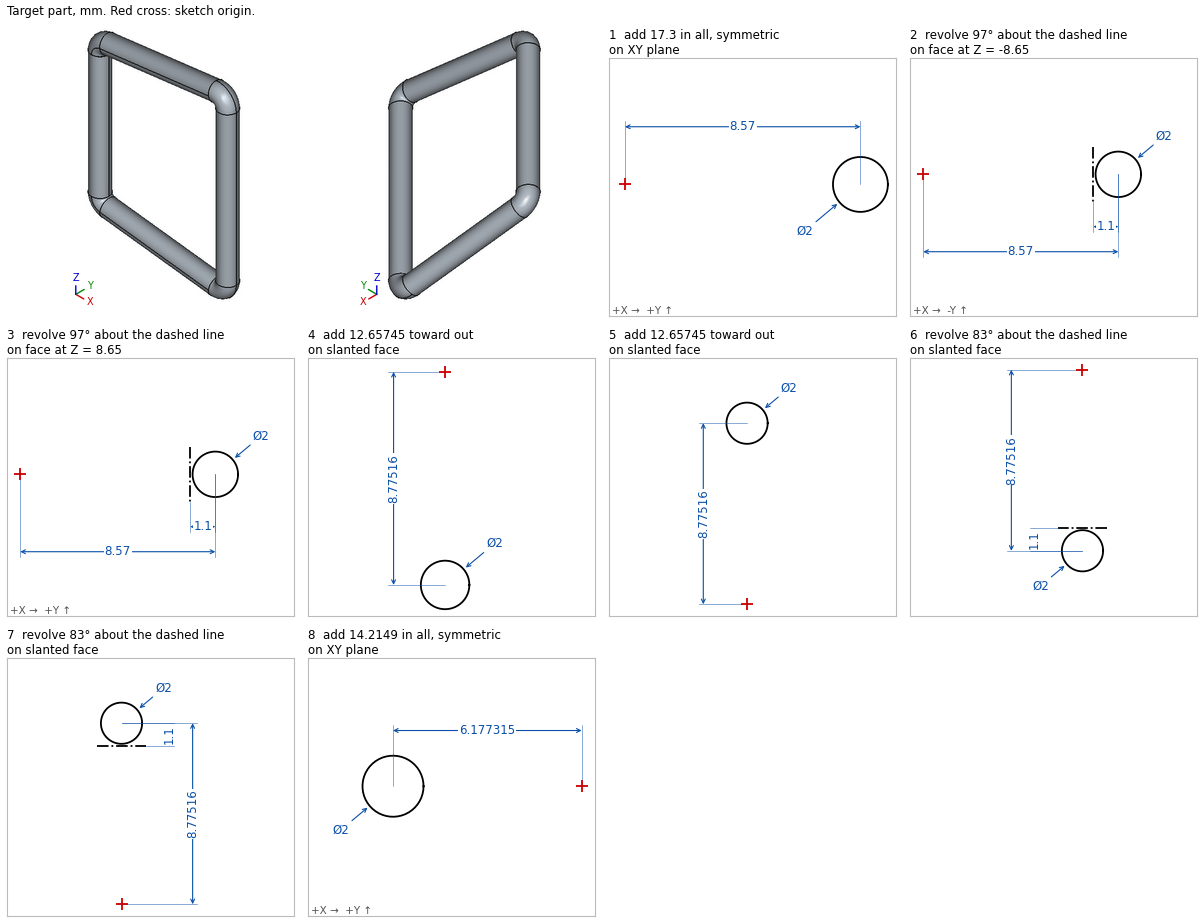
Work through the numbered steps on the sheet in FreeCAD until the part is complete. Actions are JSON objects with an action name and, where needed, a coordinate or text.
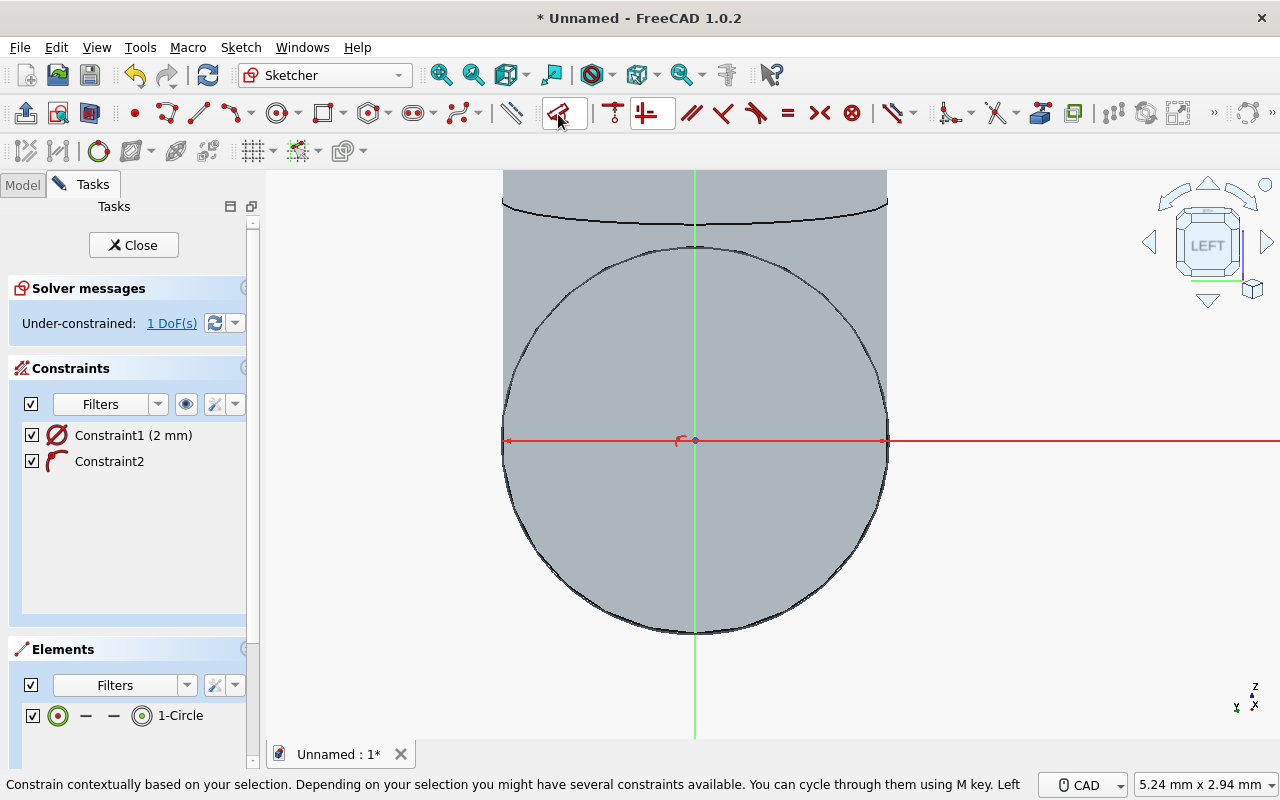
{"action": "left_click", "coordinate": [695, 441]}
{"action": "left_click", "coordinate": [661, 319]}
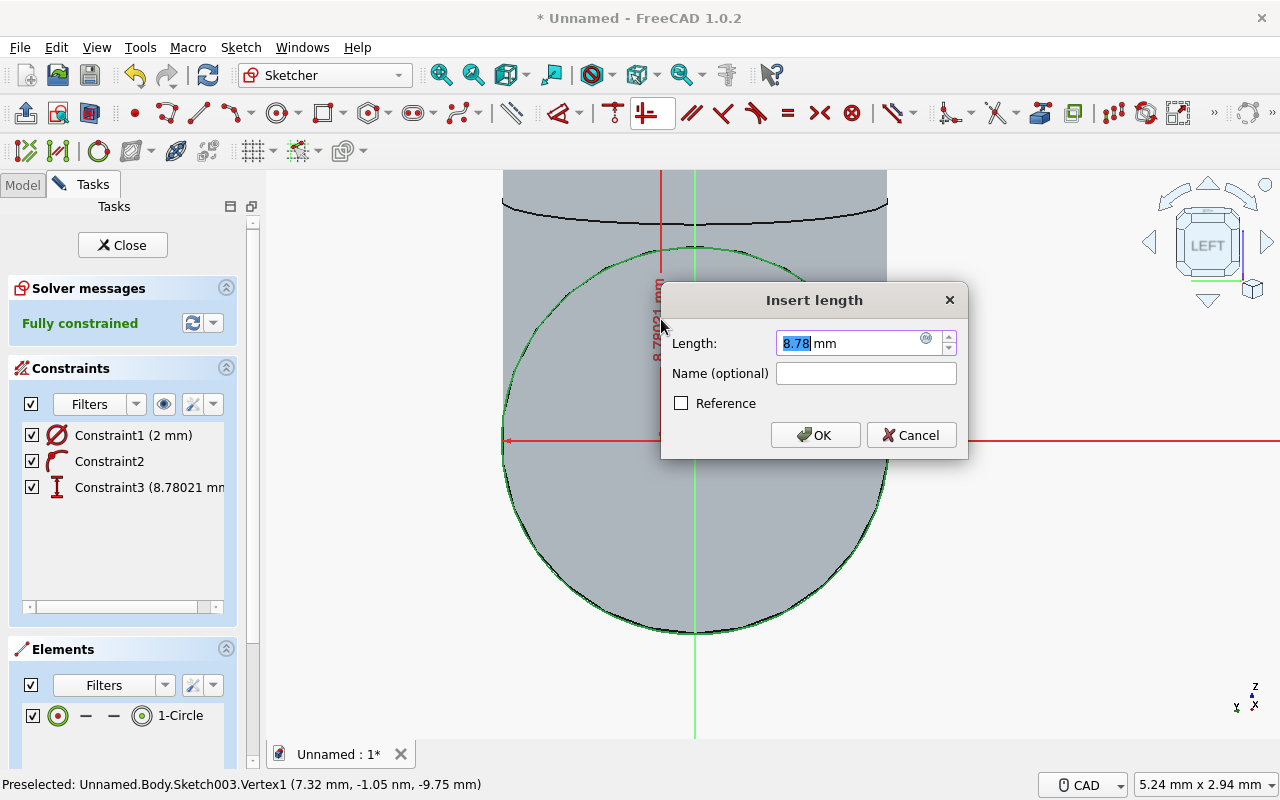
{"action": "type", "text": "8.77516"}
{"action": "key", "text": "Return"}
{"action": "key", "text": "Escape"}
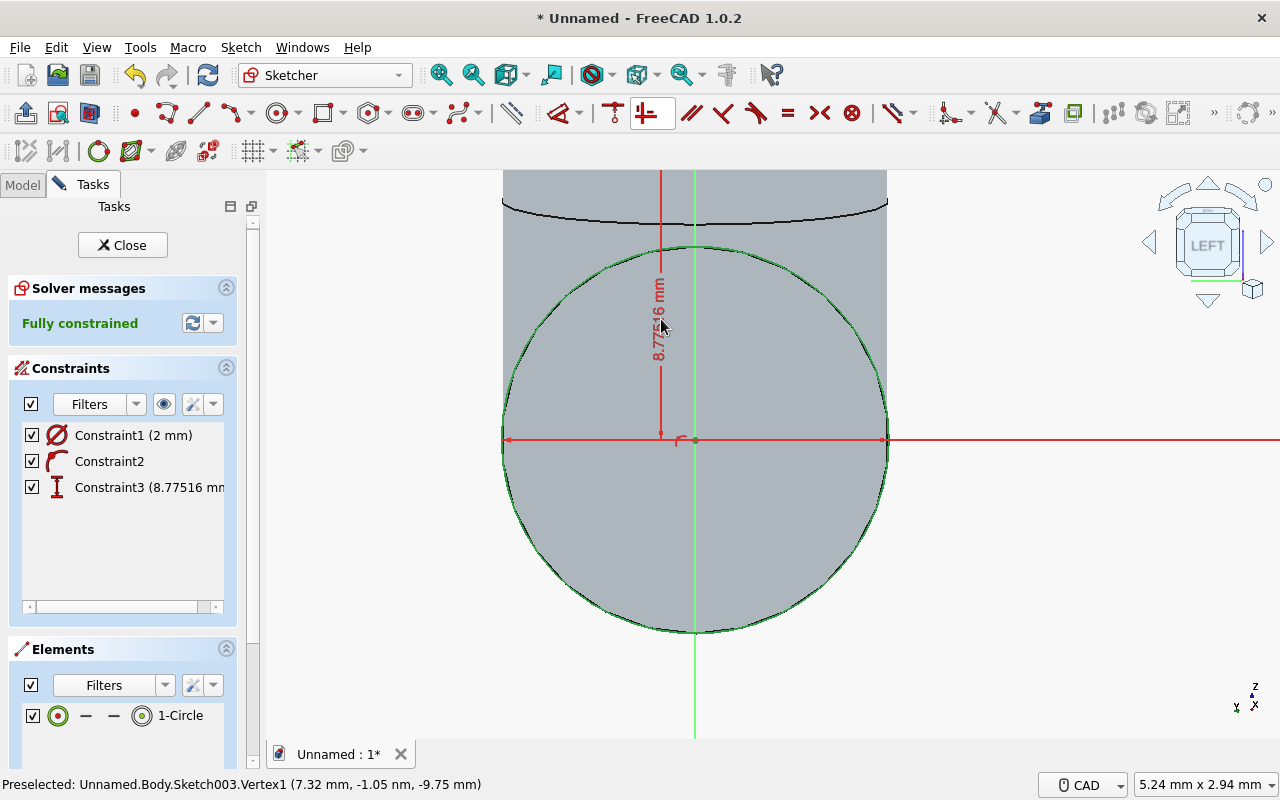
{"action": "left_click", "coordinate": [123, 245]}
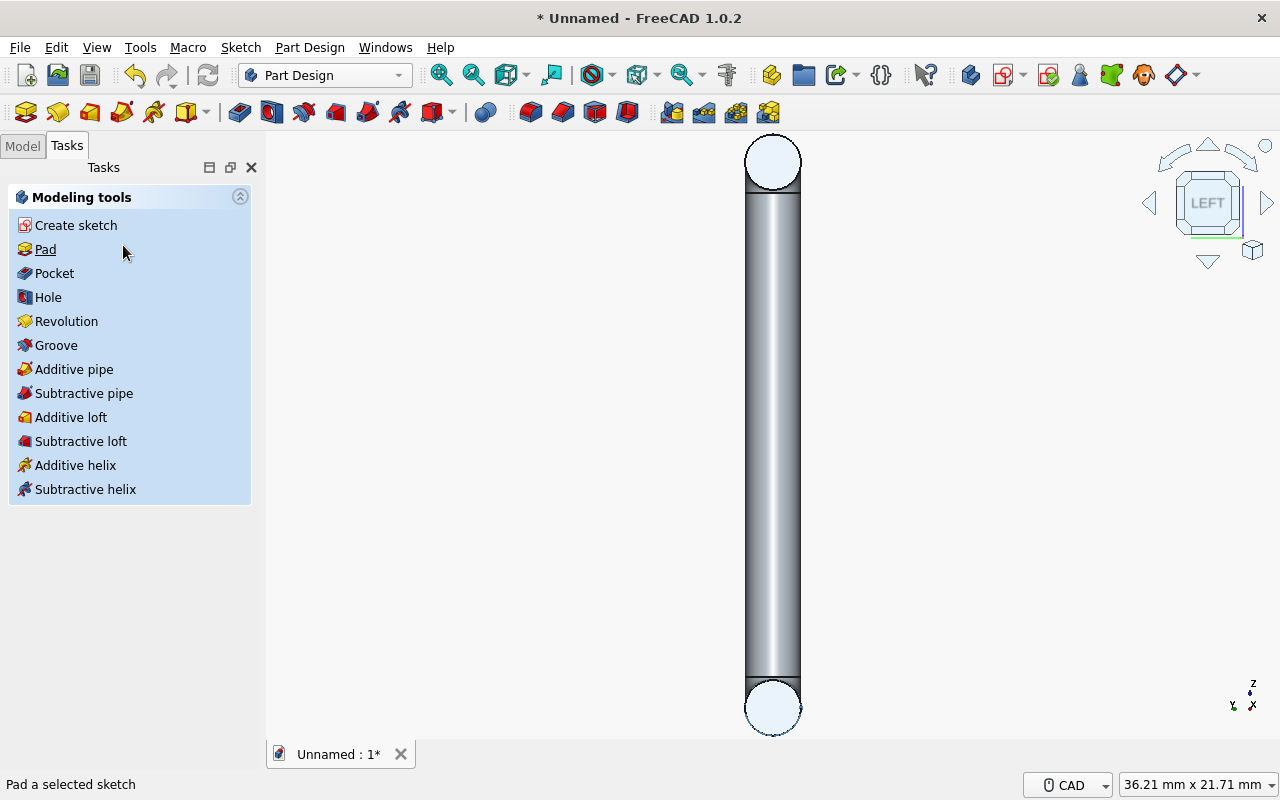
{"action": "left_click", "coordinate": [26, 112]}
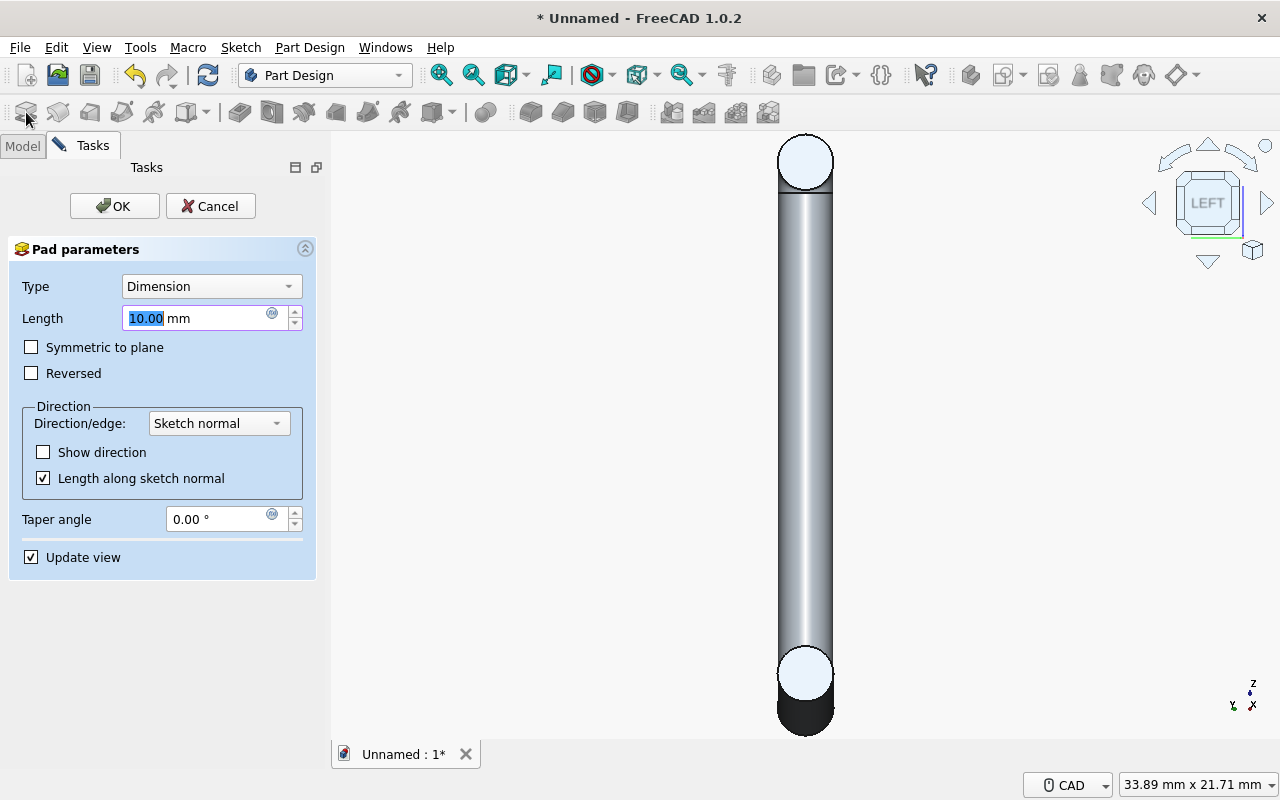
{"action": "type", "text": "12.65745"}
{"action": "key", "text": "Tab"}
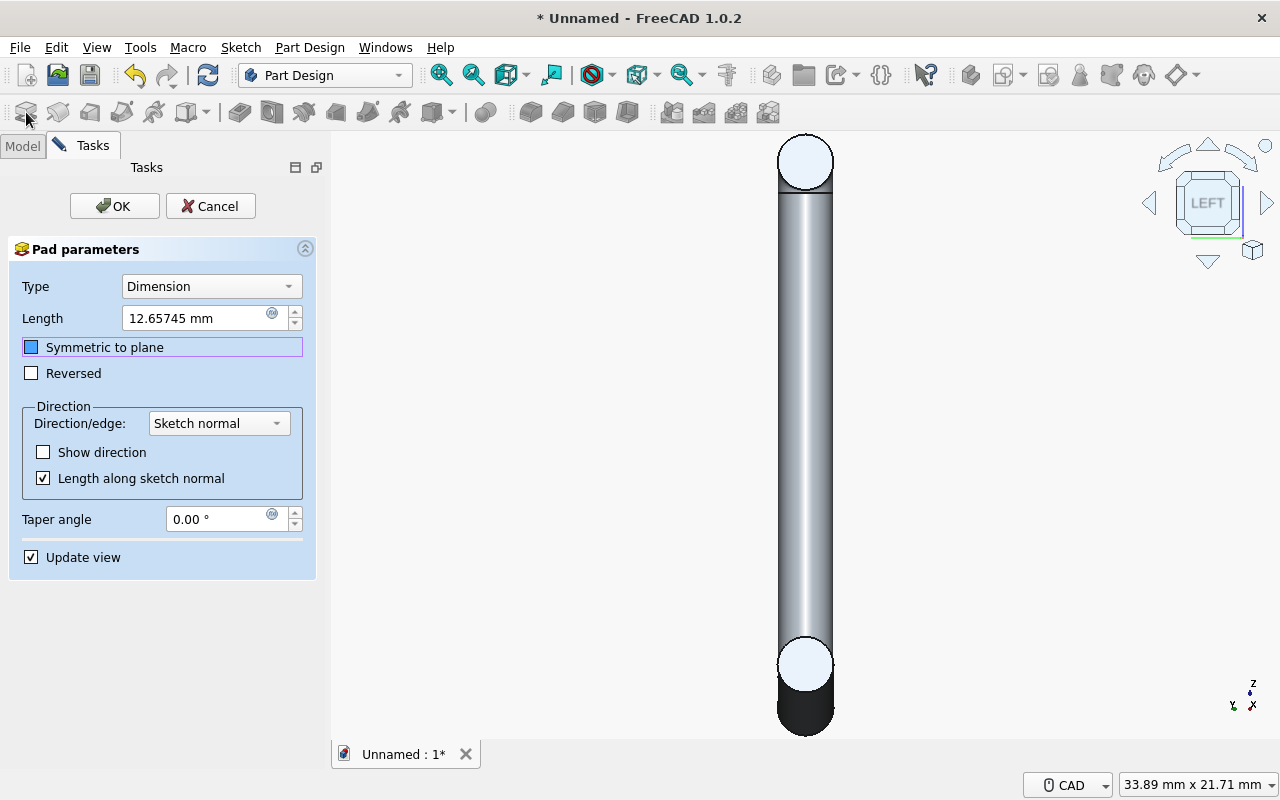
{"action": "left_click", "coordinate": [115, 206]}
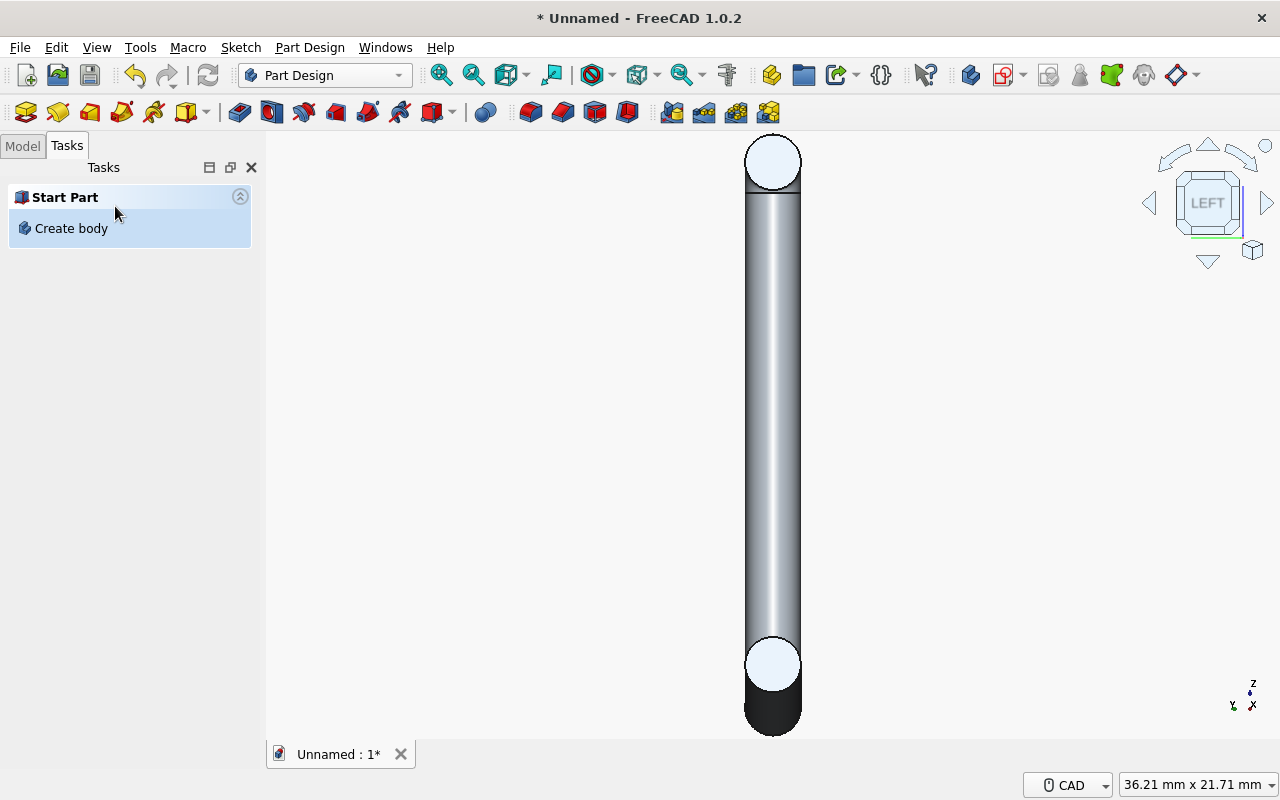
{"action": "left_click", "coordinate": [773, 161]}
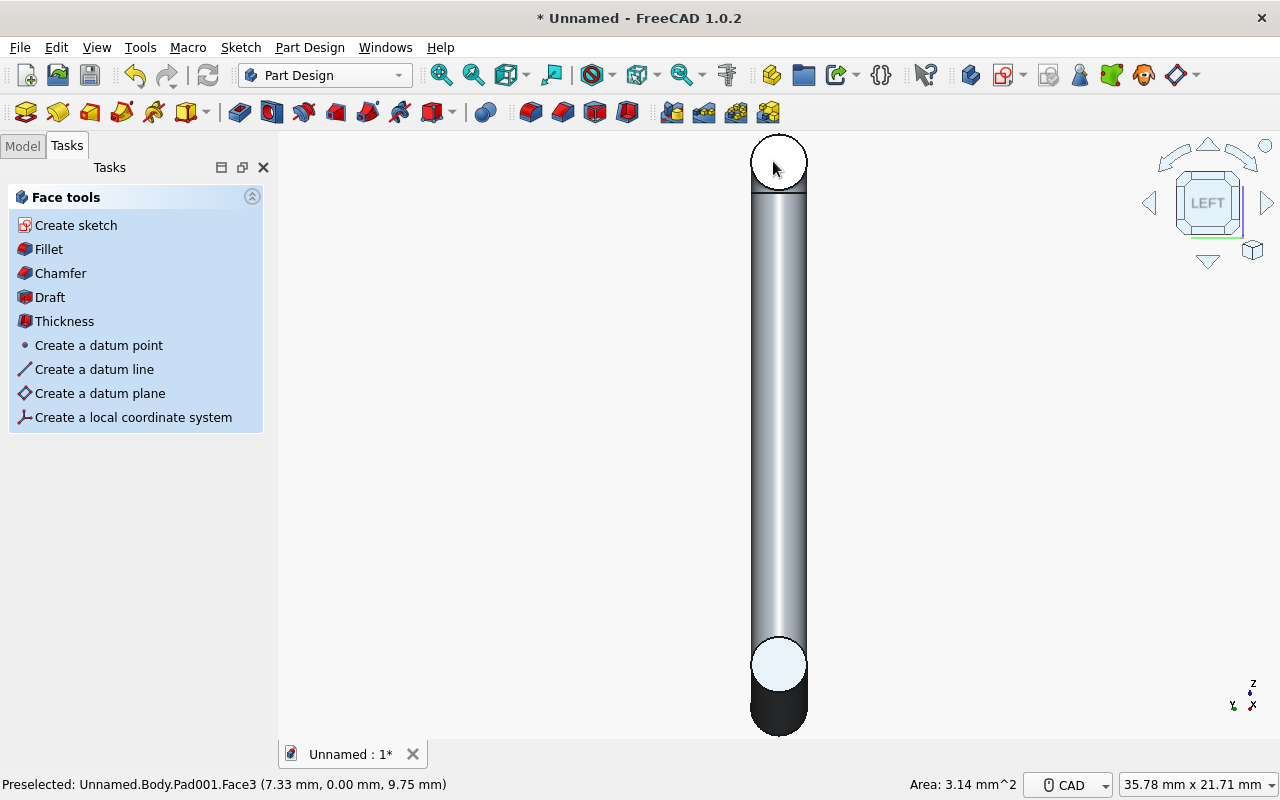
{"action": "left_click", "coordinate": [1004, 76]}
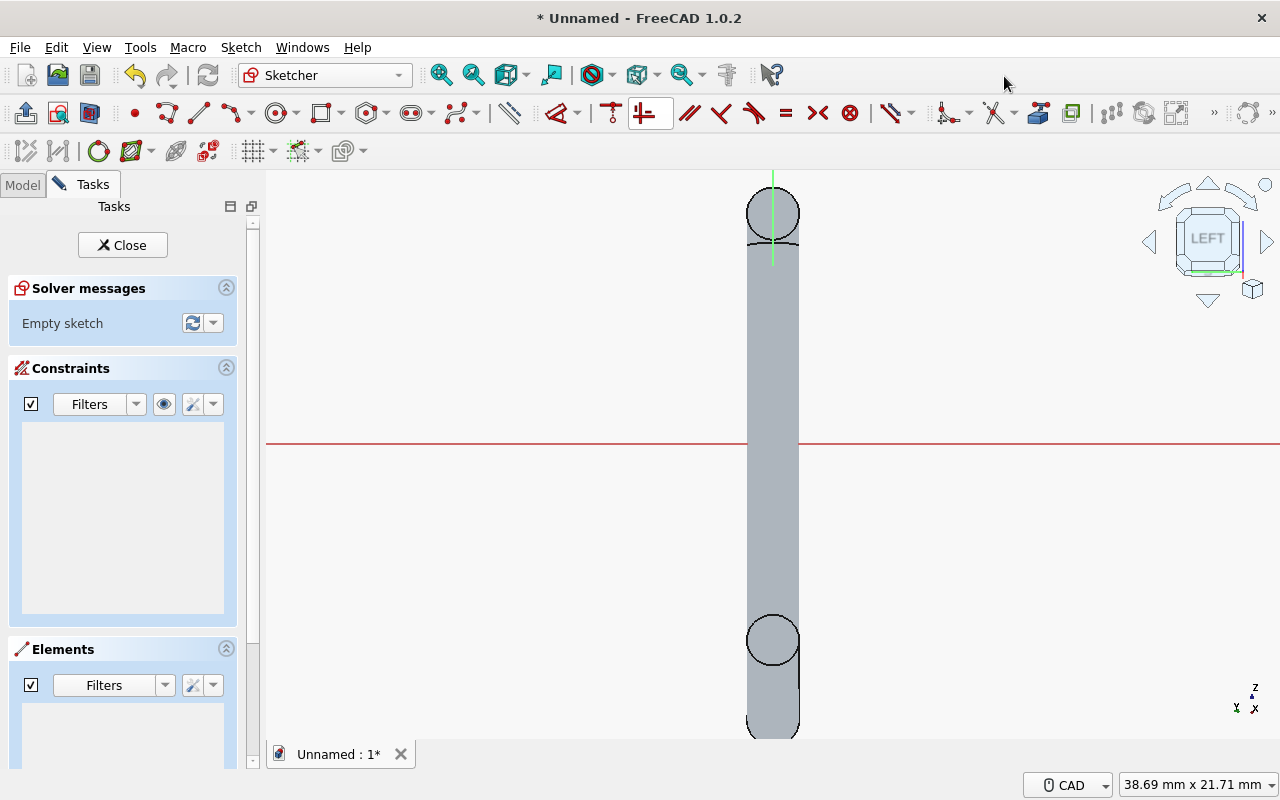
{"action": "scroll", "coordinate": [704, 454], "scroll_direction": "down", "scroll_amount": 5}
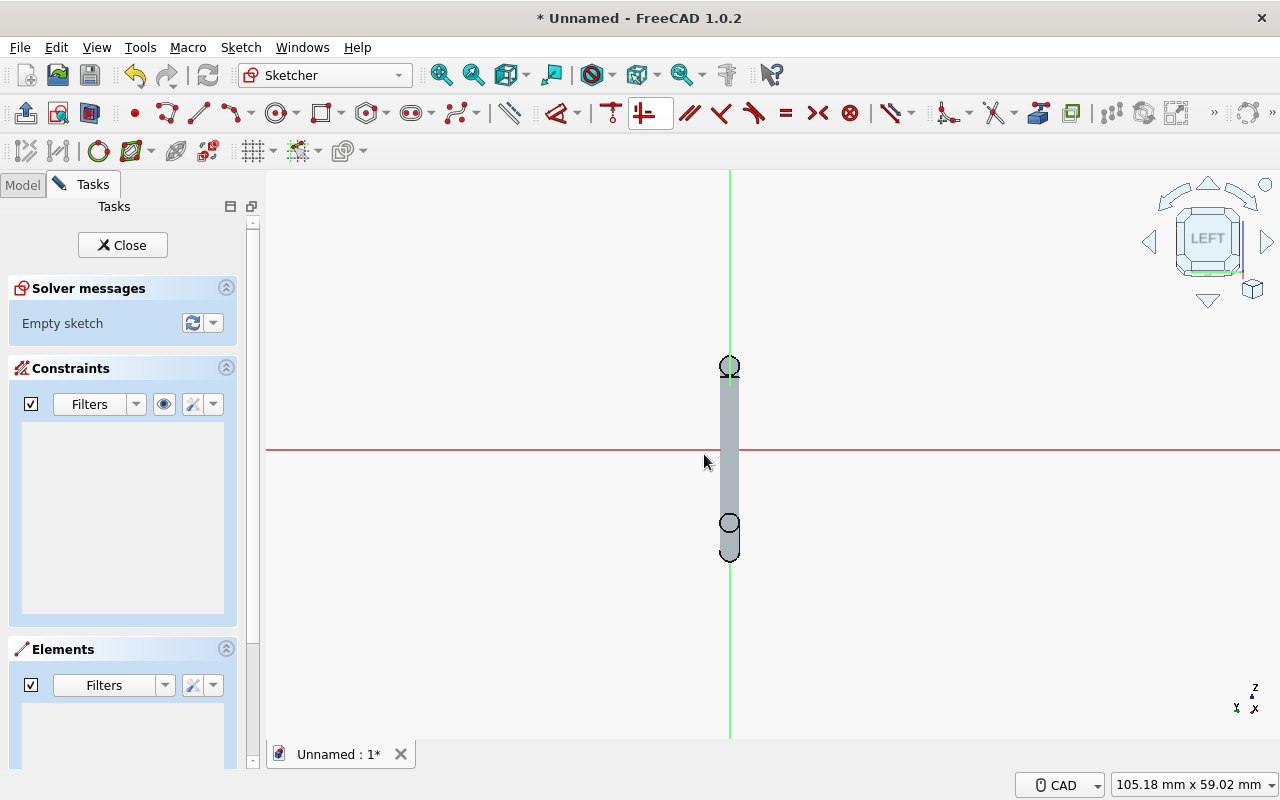
{"action": "scroll", "coordinate": [731, 361], "scroll_direction": "up", "scroll_amount": 15}